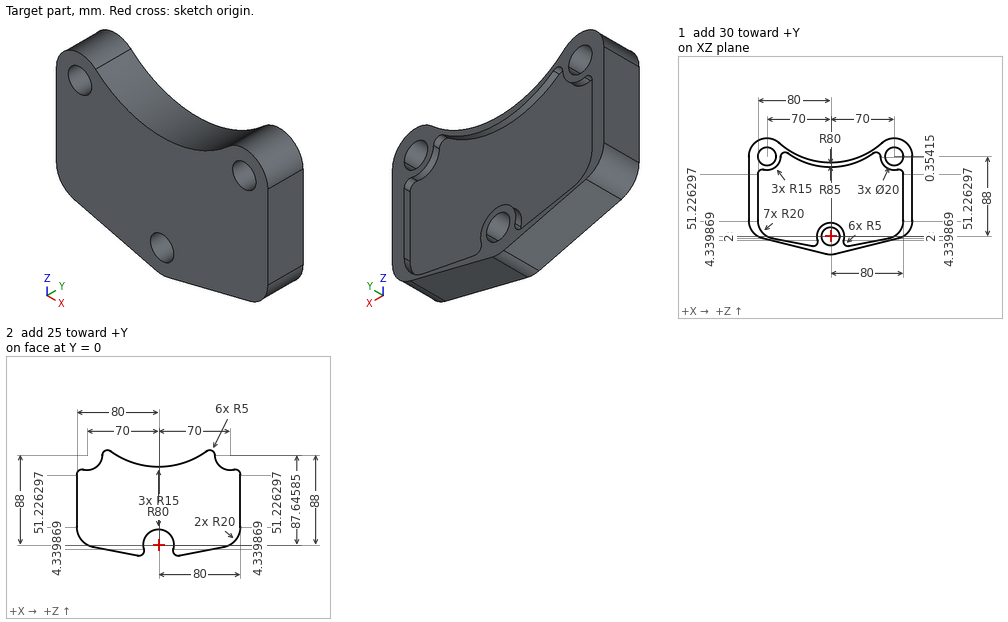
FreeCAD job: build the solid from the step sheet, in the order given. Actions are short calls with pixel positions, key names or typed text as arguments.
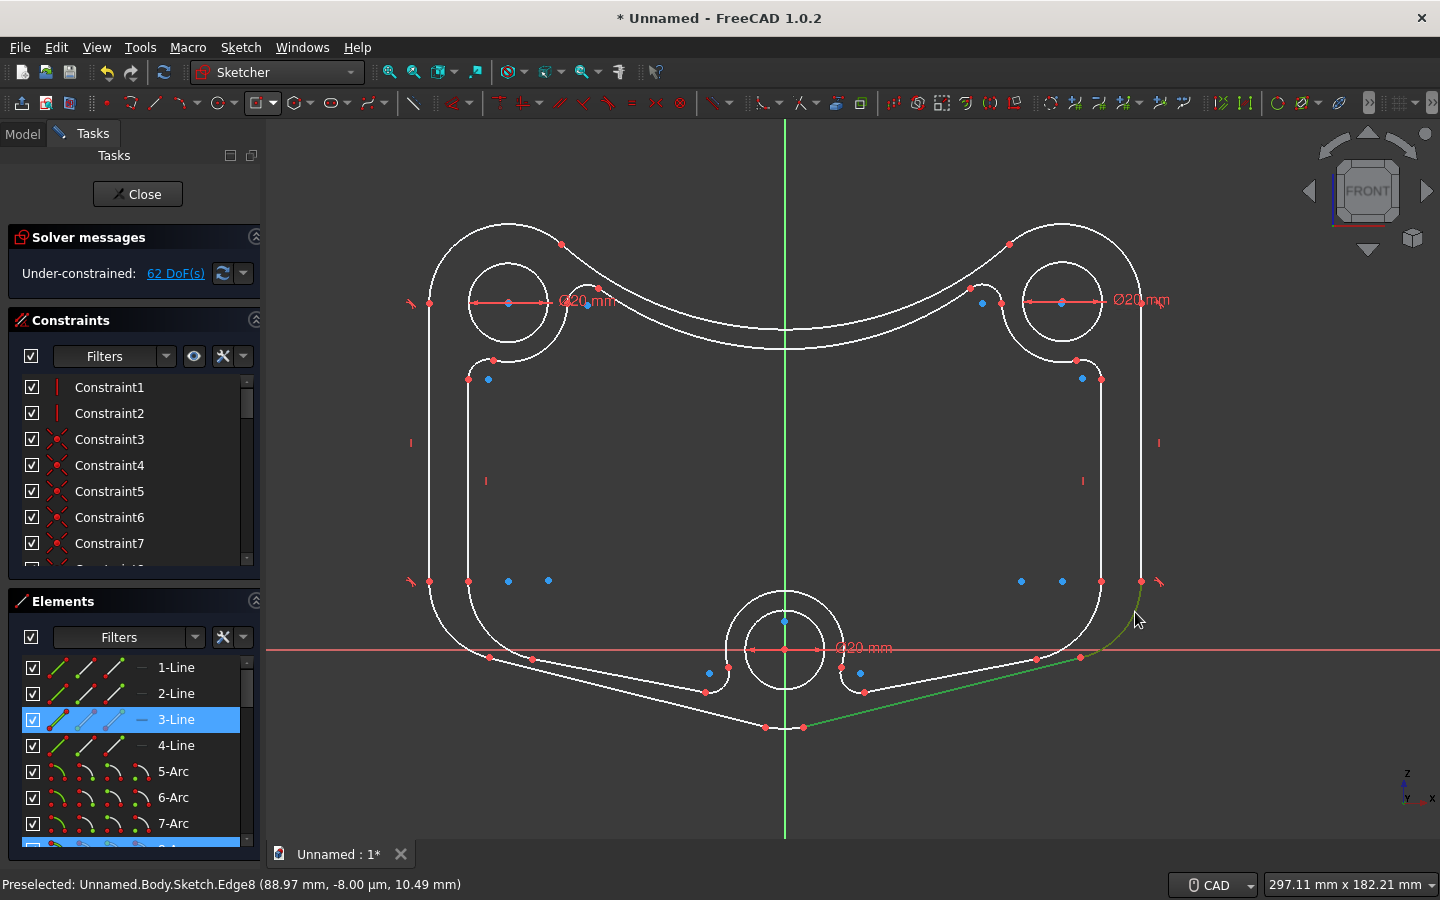
key(t)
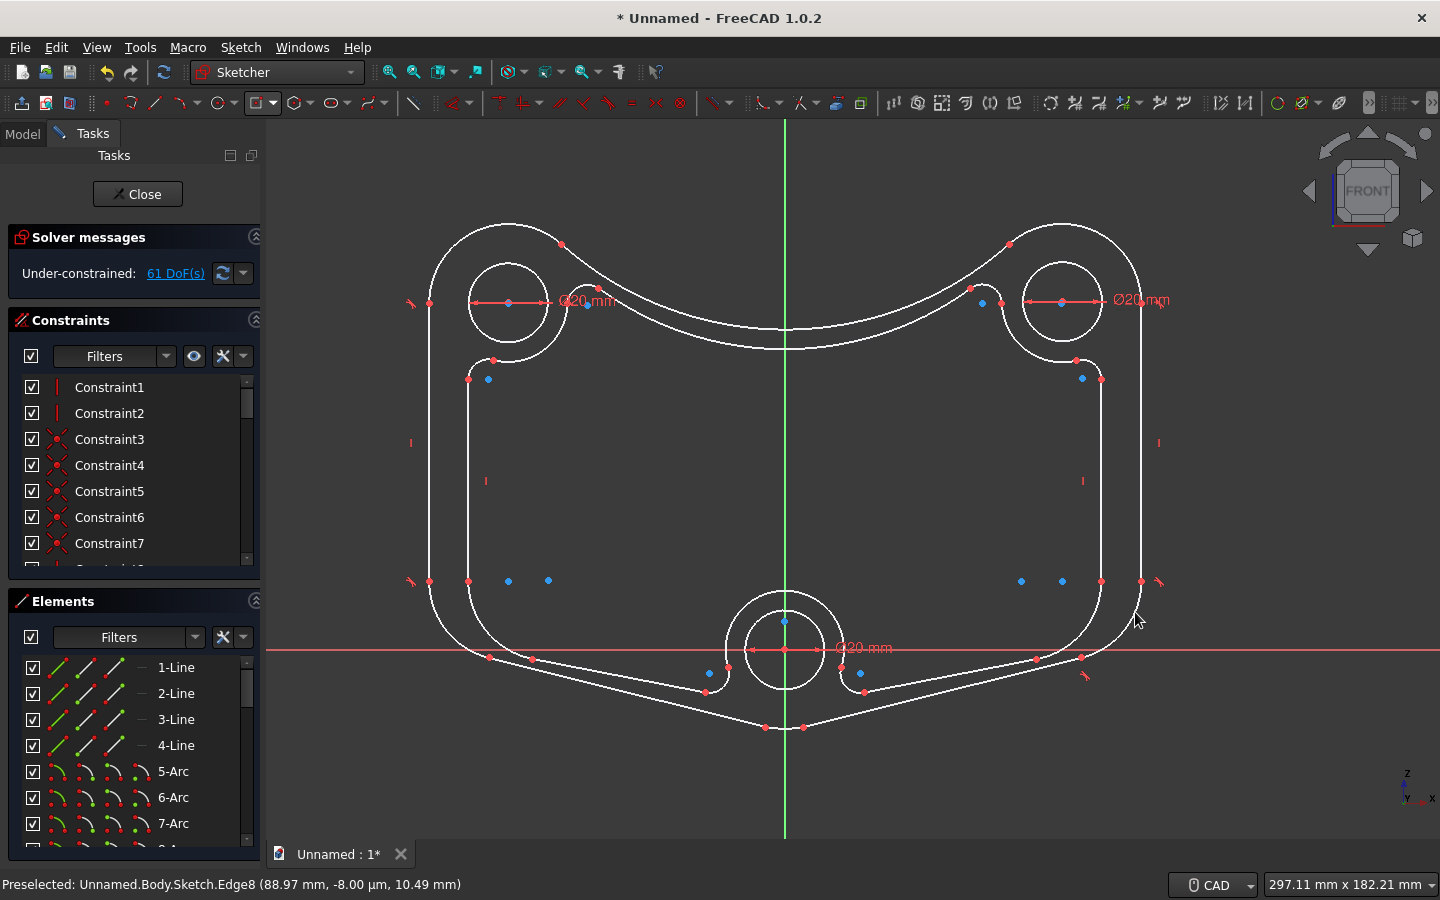
click(998, 679)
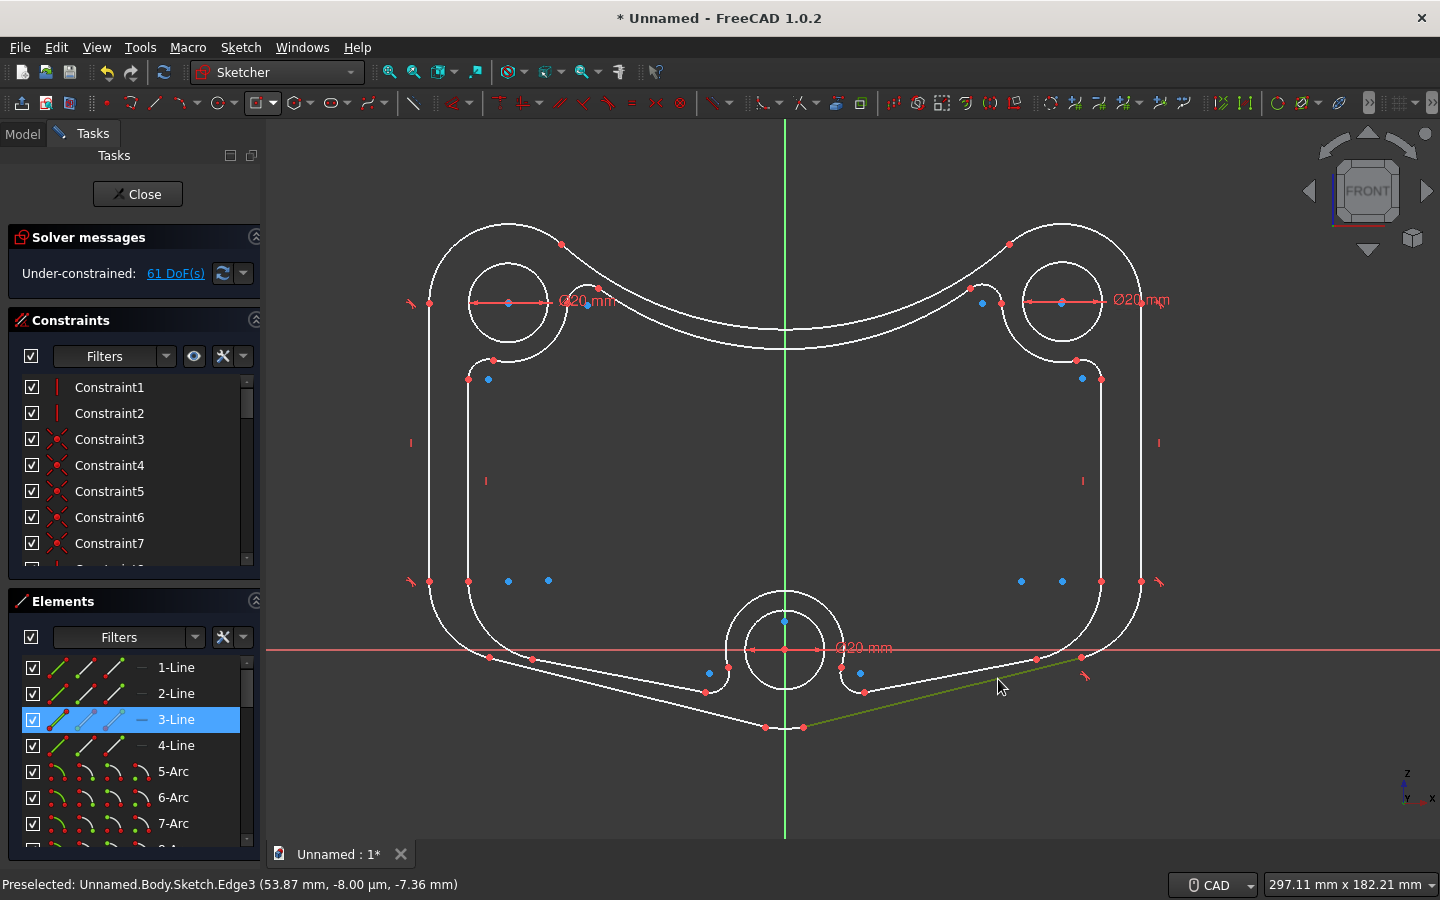
click(785, 729)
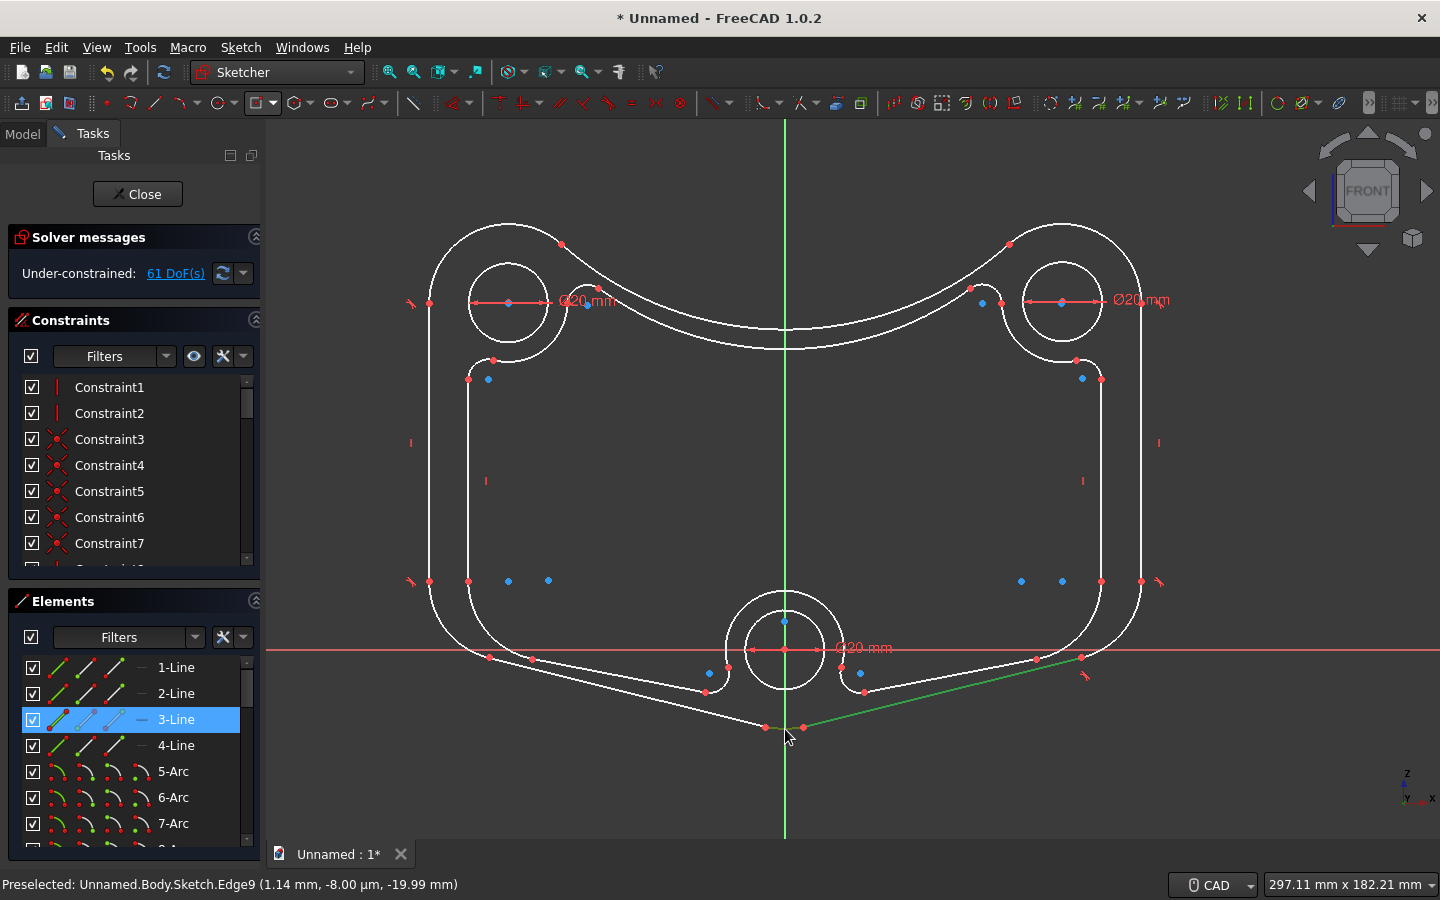
click(608, 104)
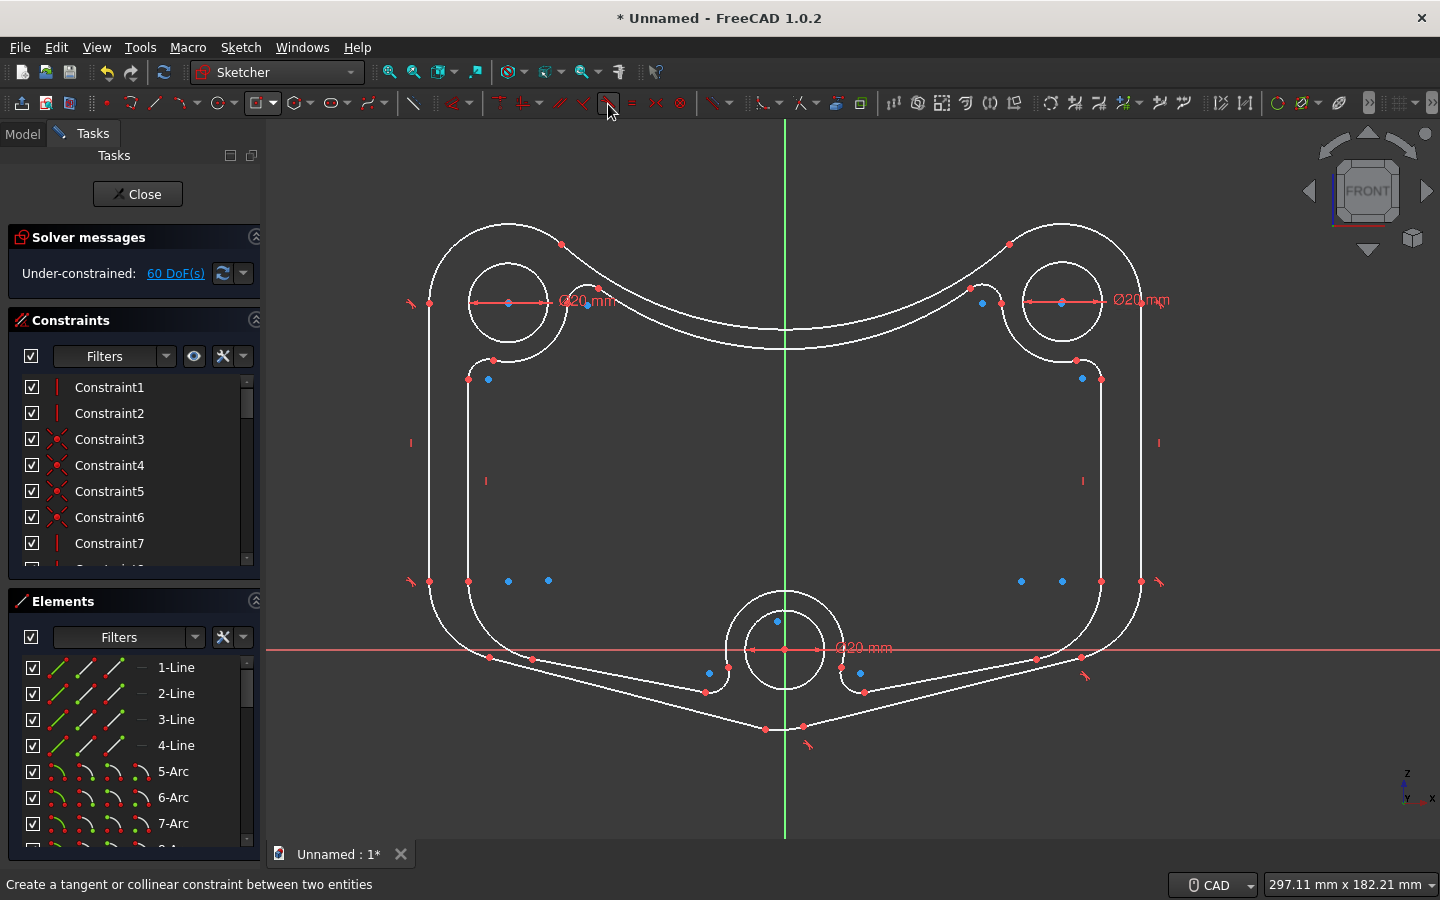
click(683, 708)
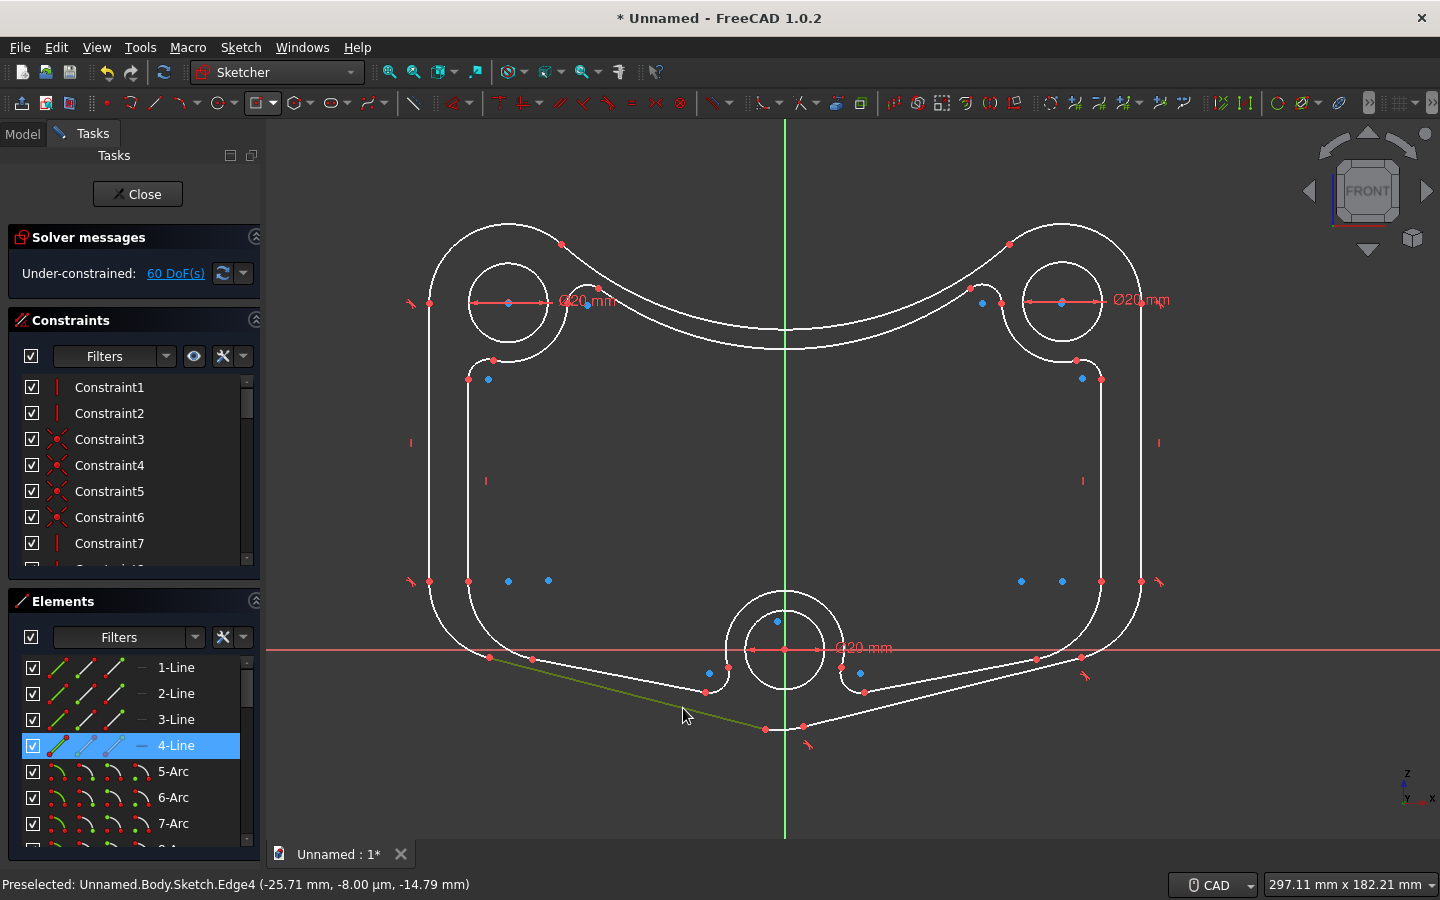
click(785, 730)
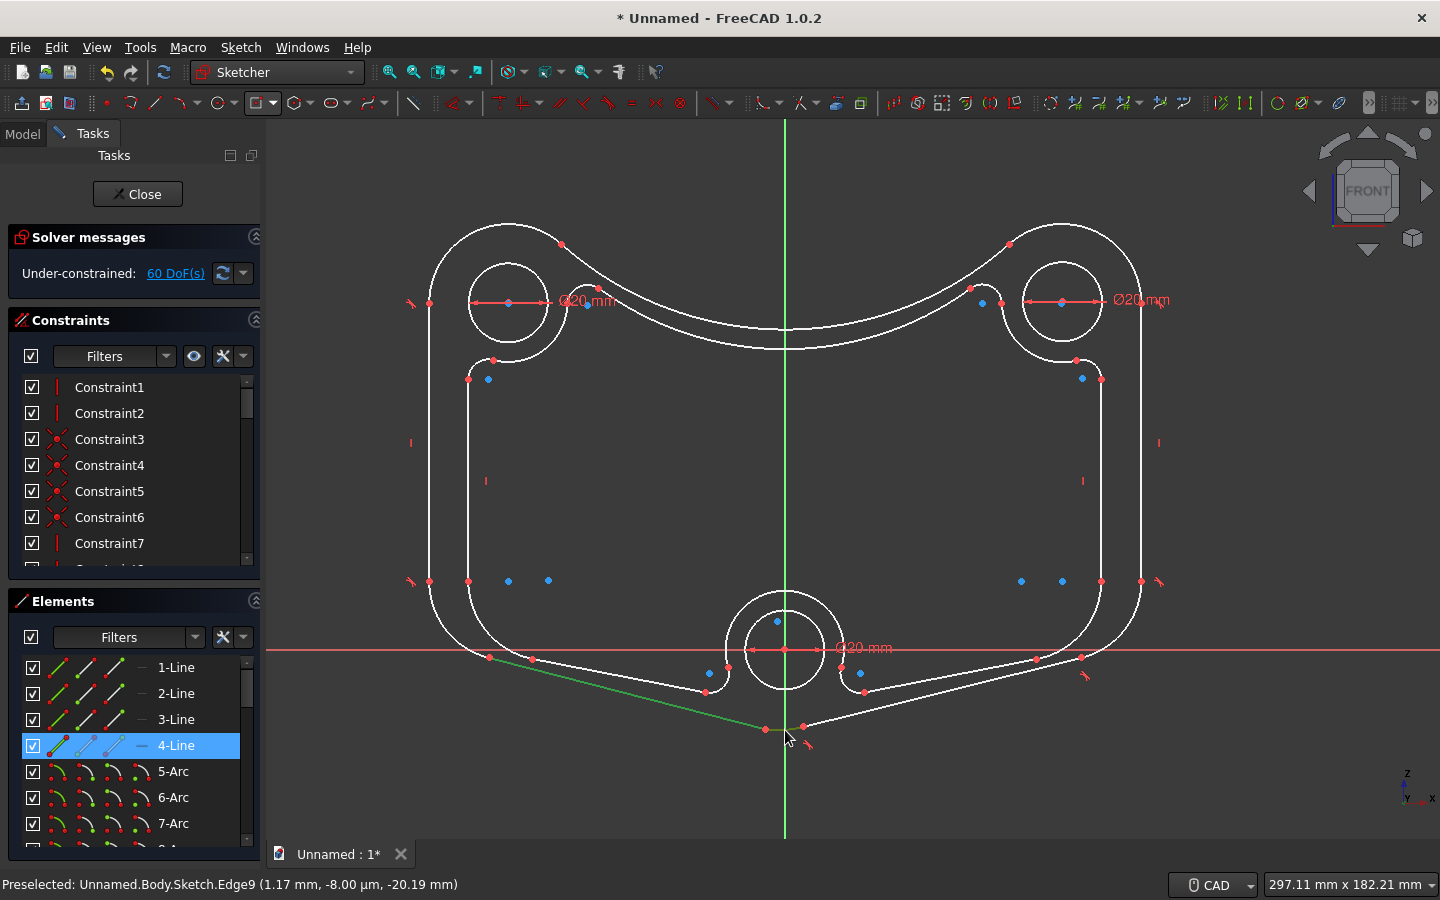
key(t)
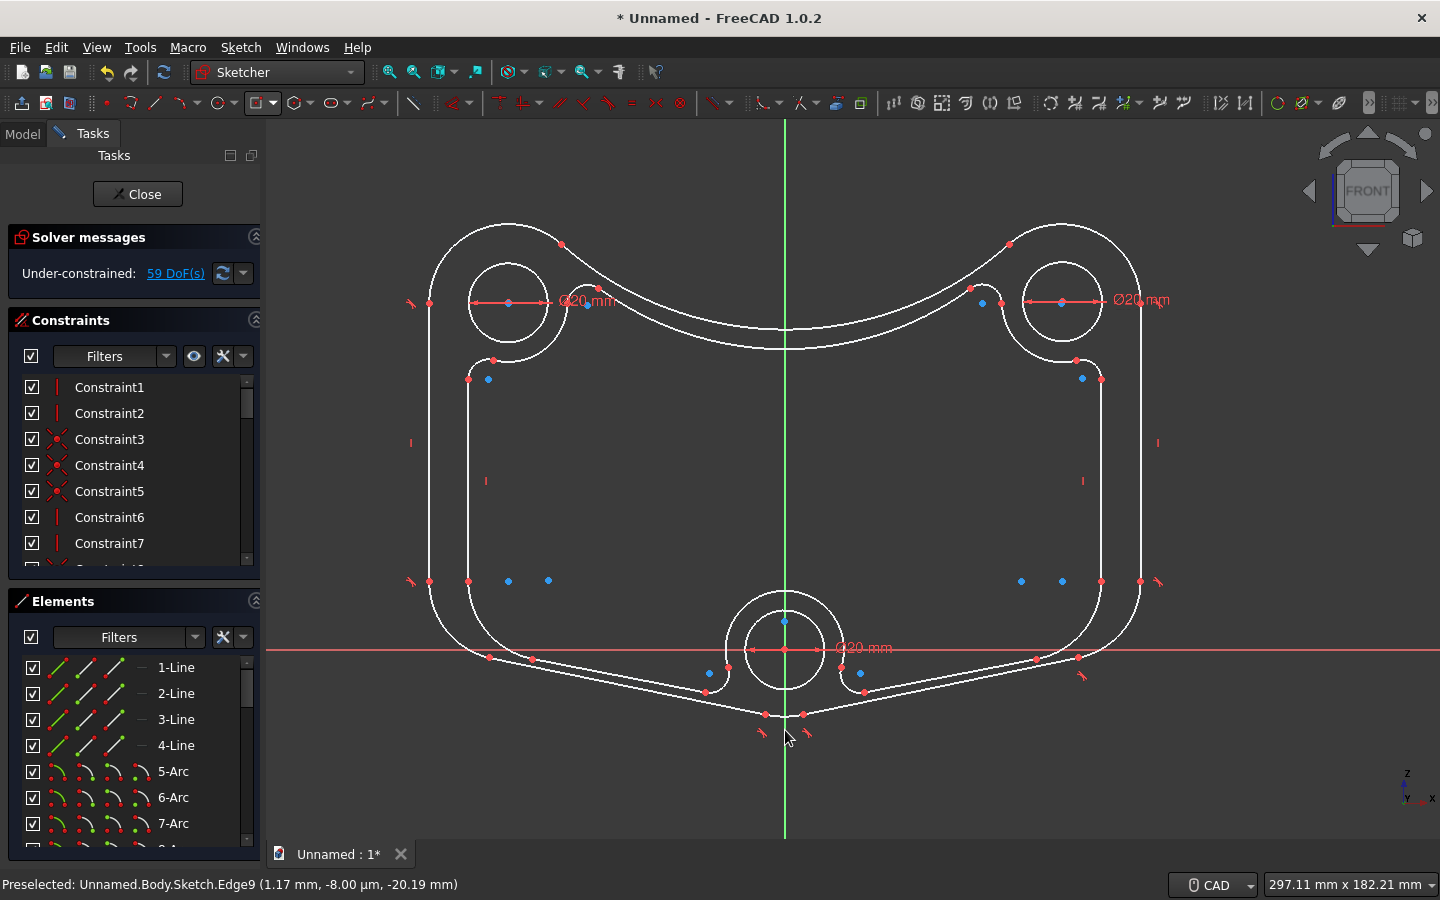
scroll(683, 698, up, 2)